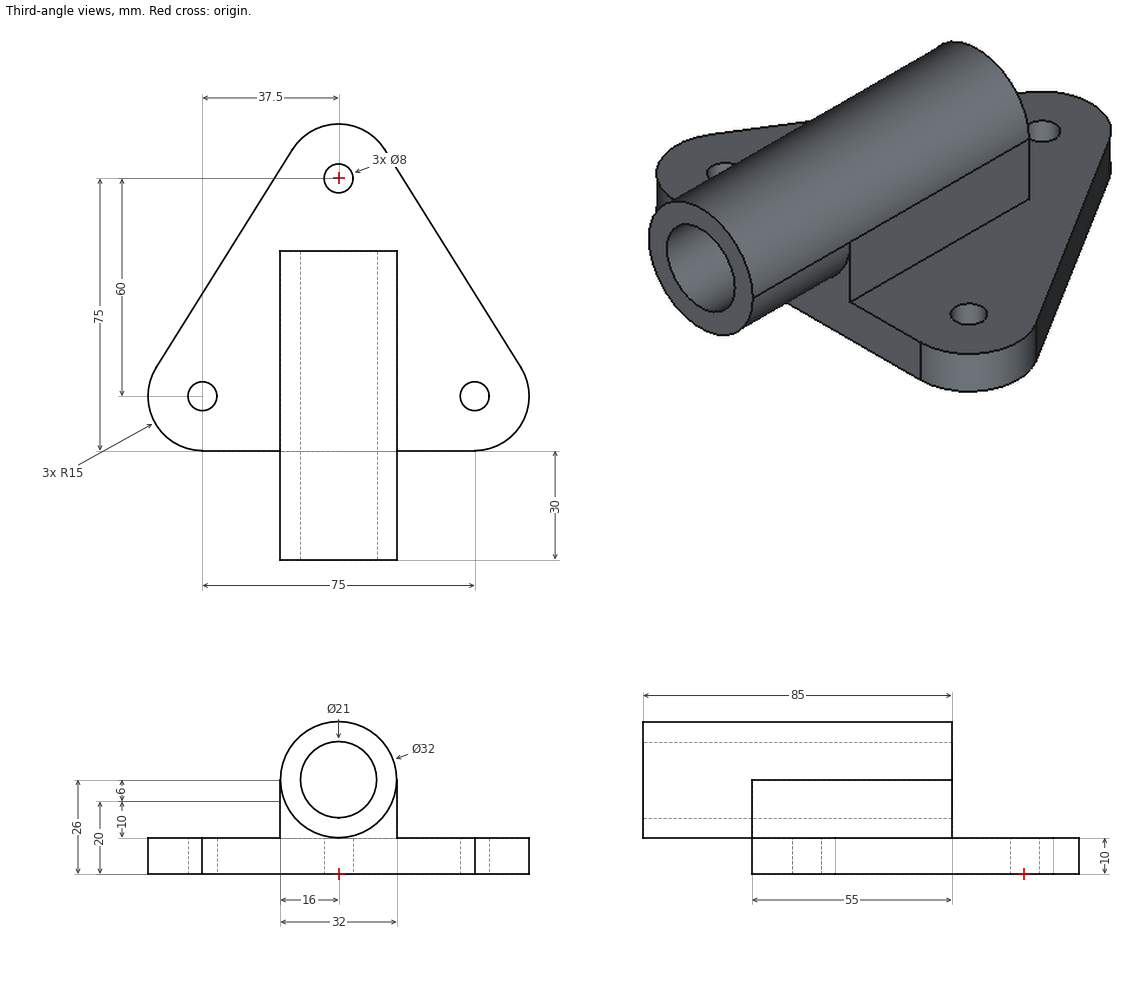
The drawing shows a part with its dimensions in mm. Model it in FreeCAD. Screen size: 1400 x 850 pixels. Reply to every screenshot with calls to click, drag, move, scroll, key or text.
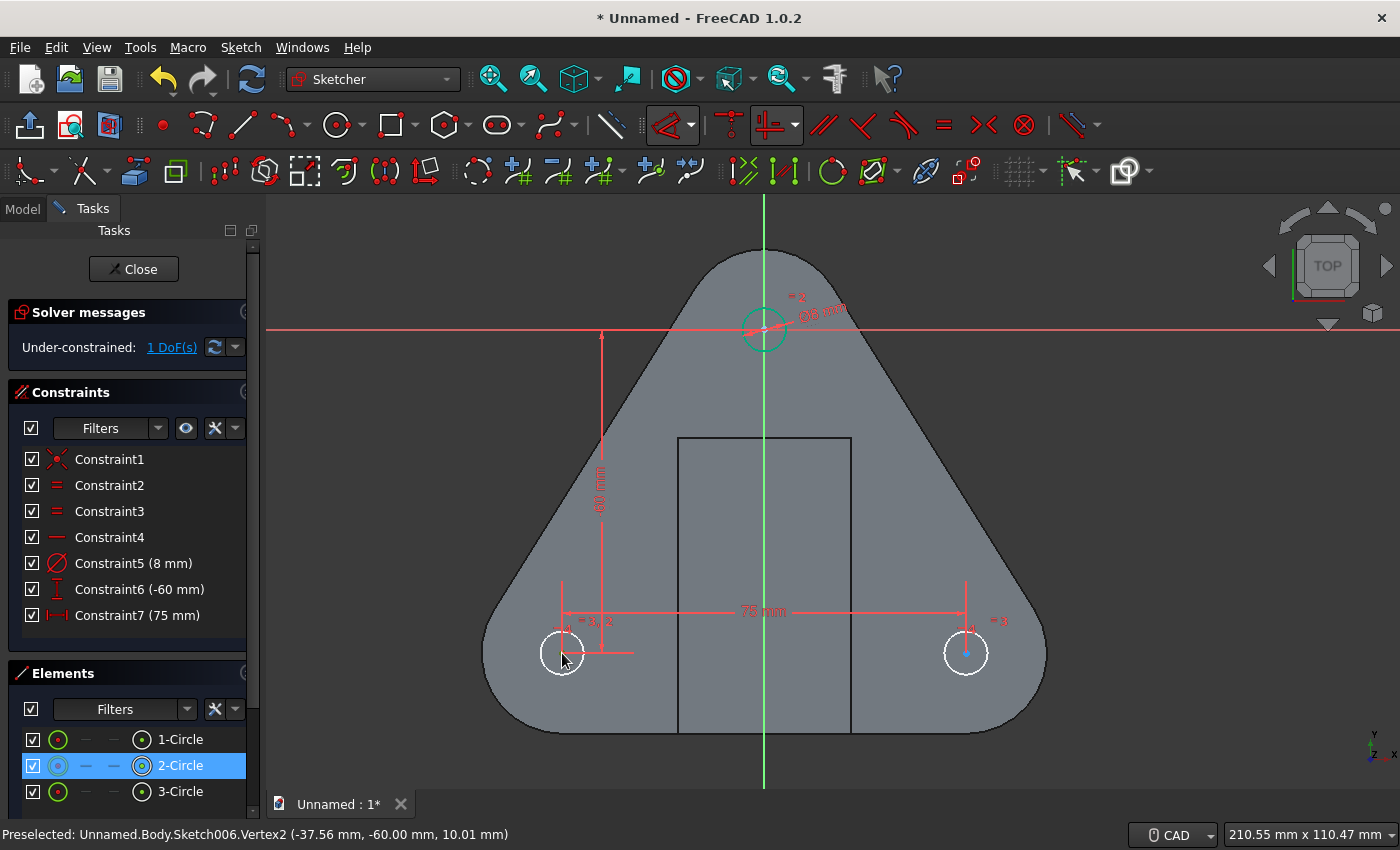
key(l)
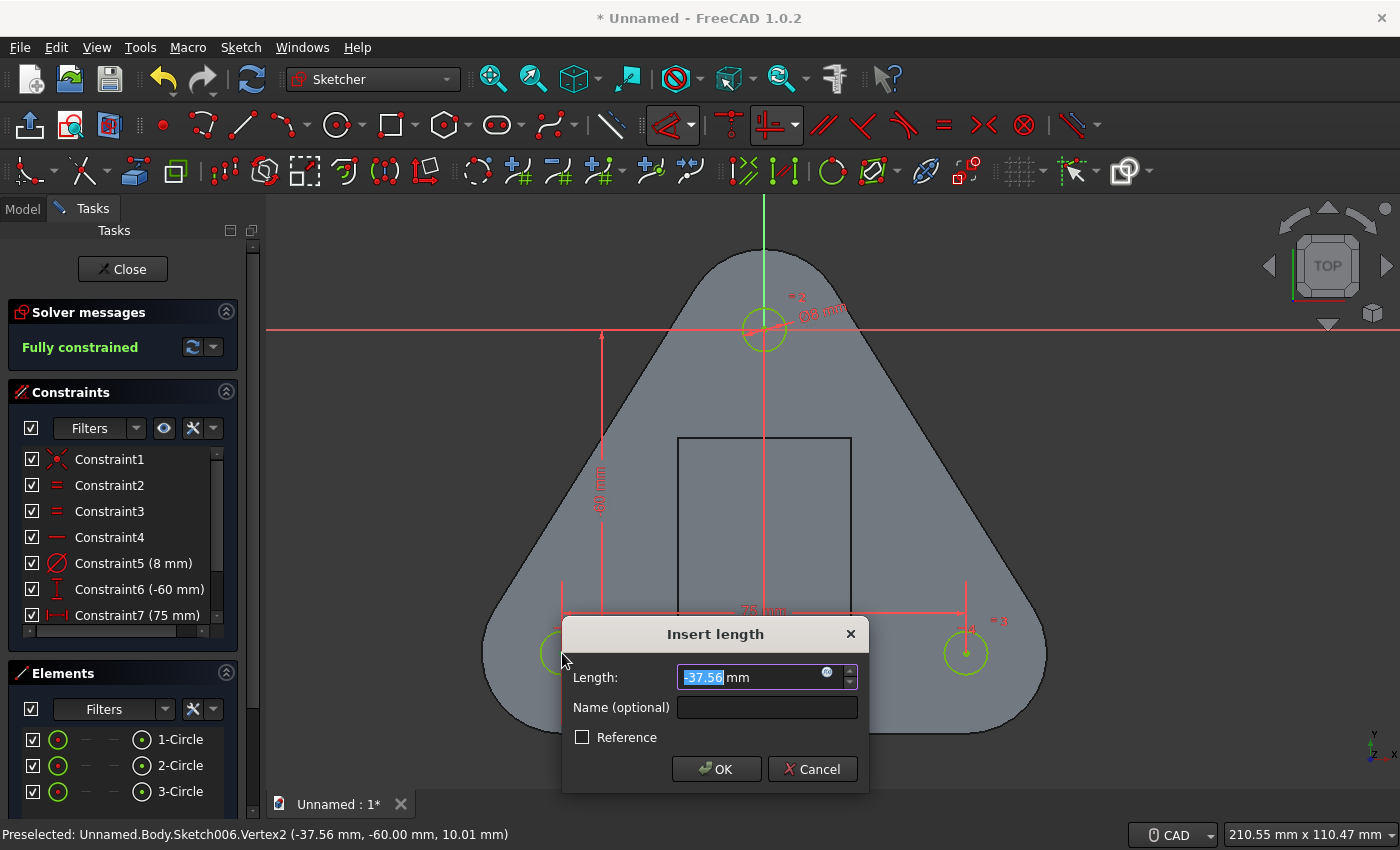
text(-37.5)
key(Return)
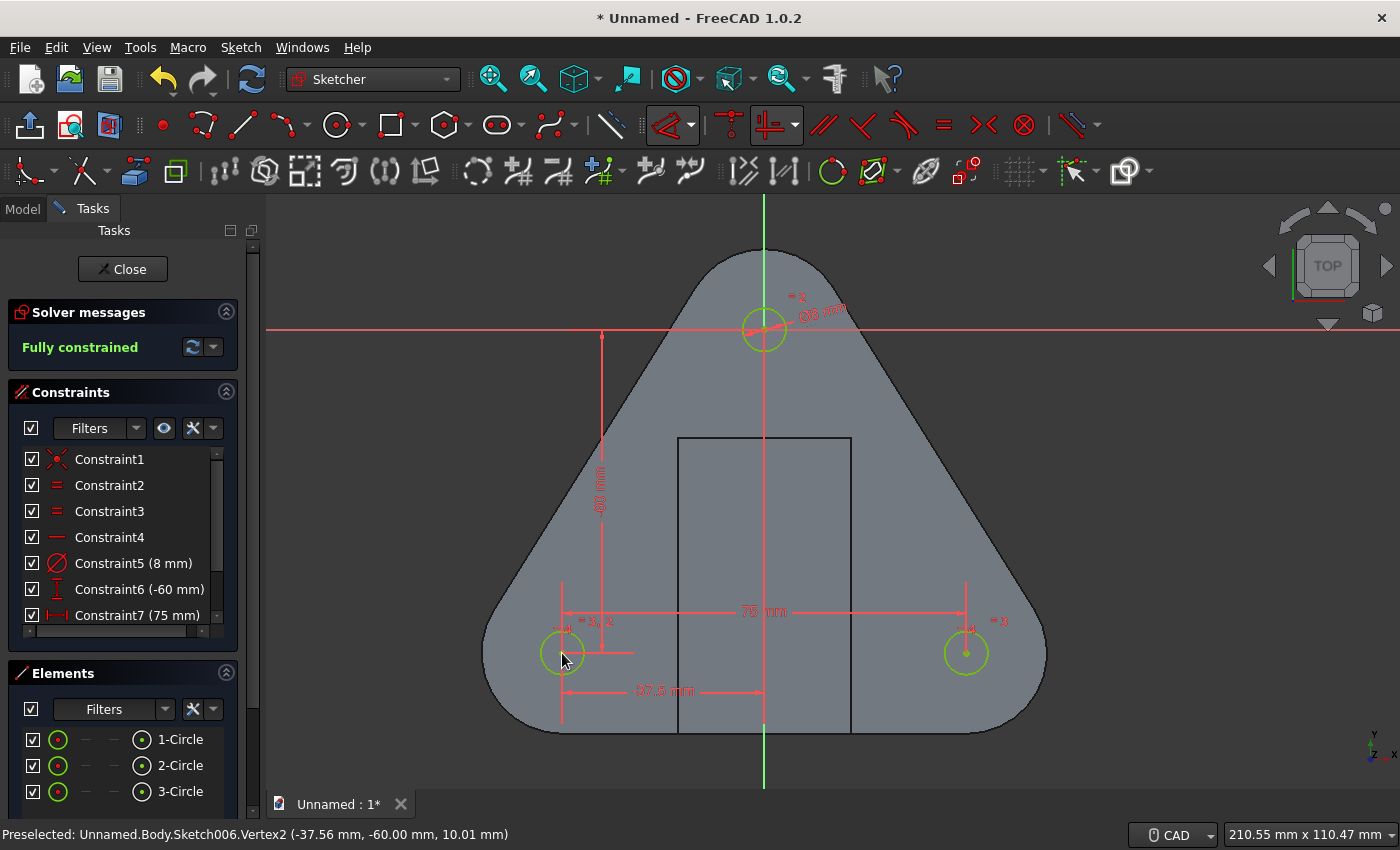
click(123, 269)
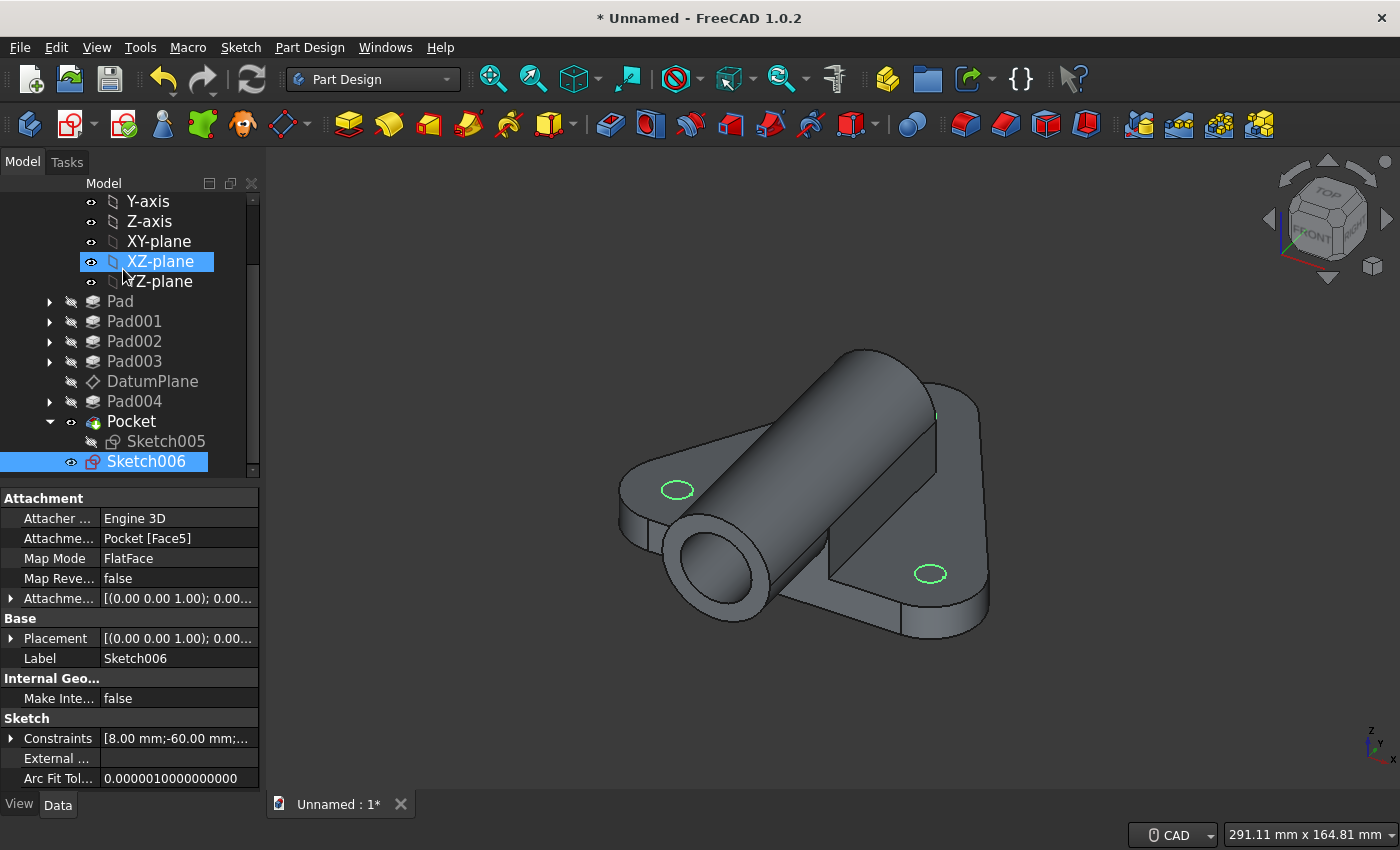
click(612, 124)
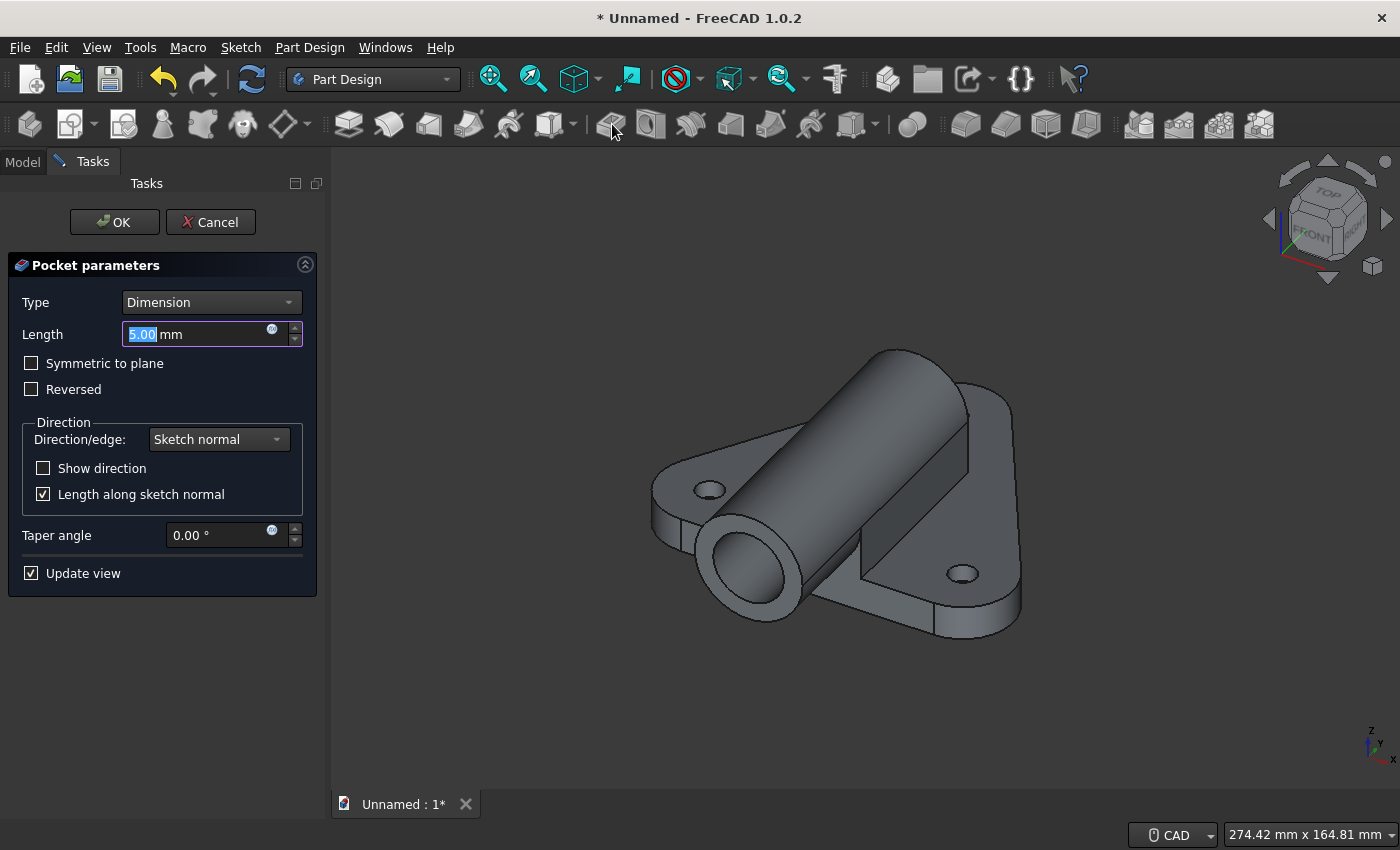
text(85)
key(Tab)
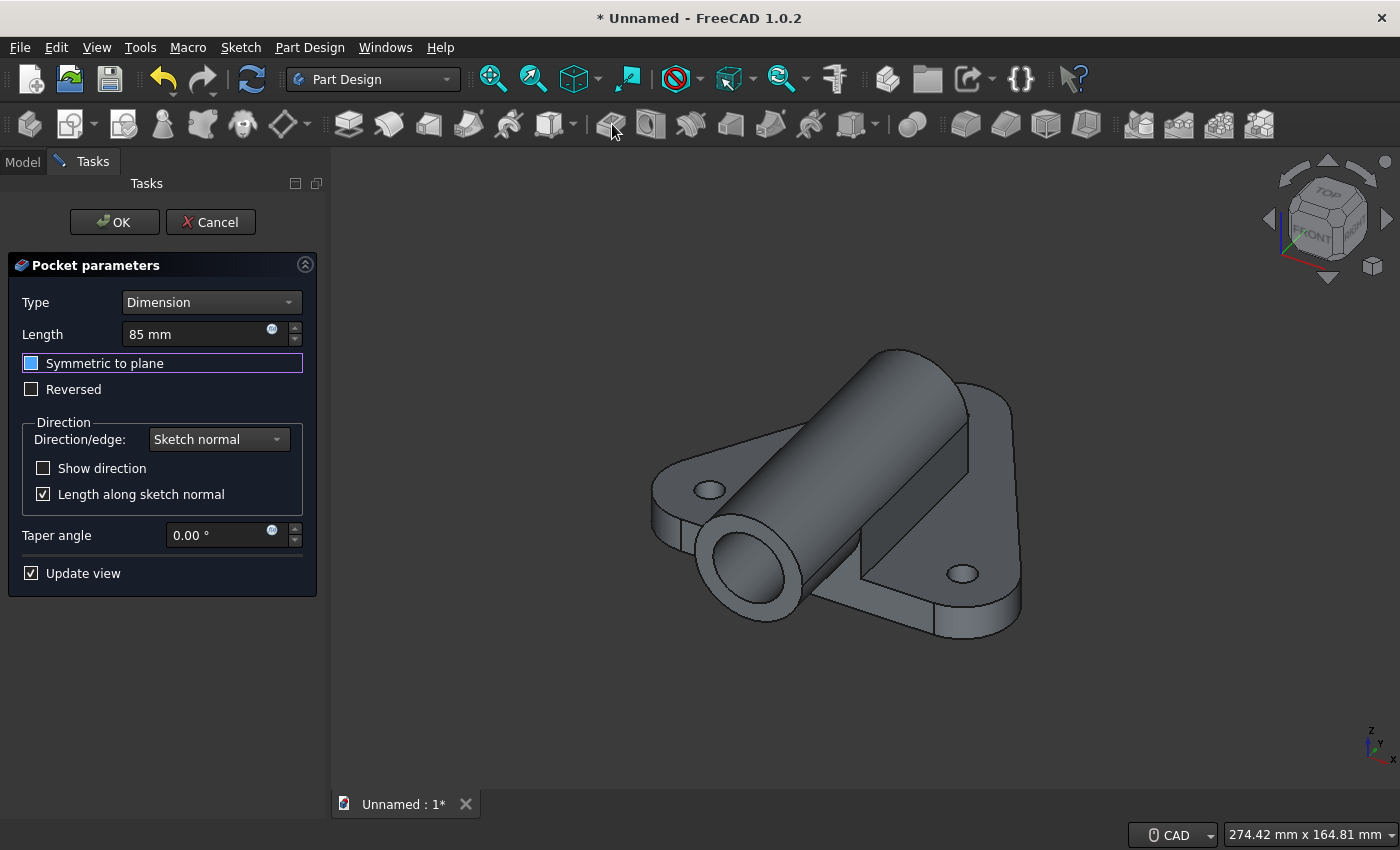
click(115, 222)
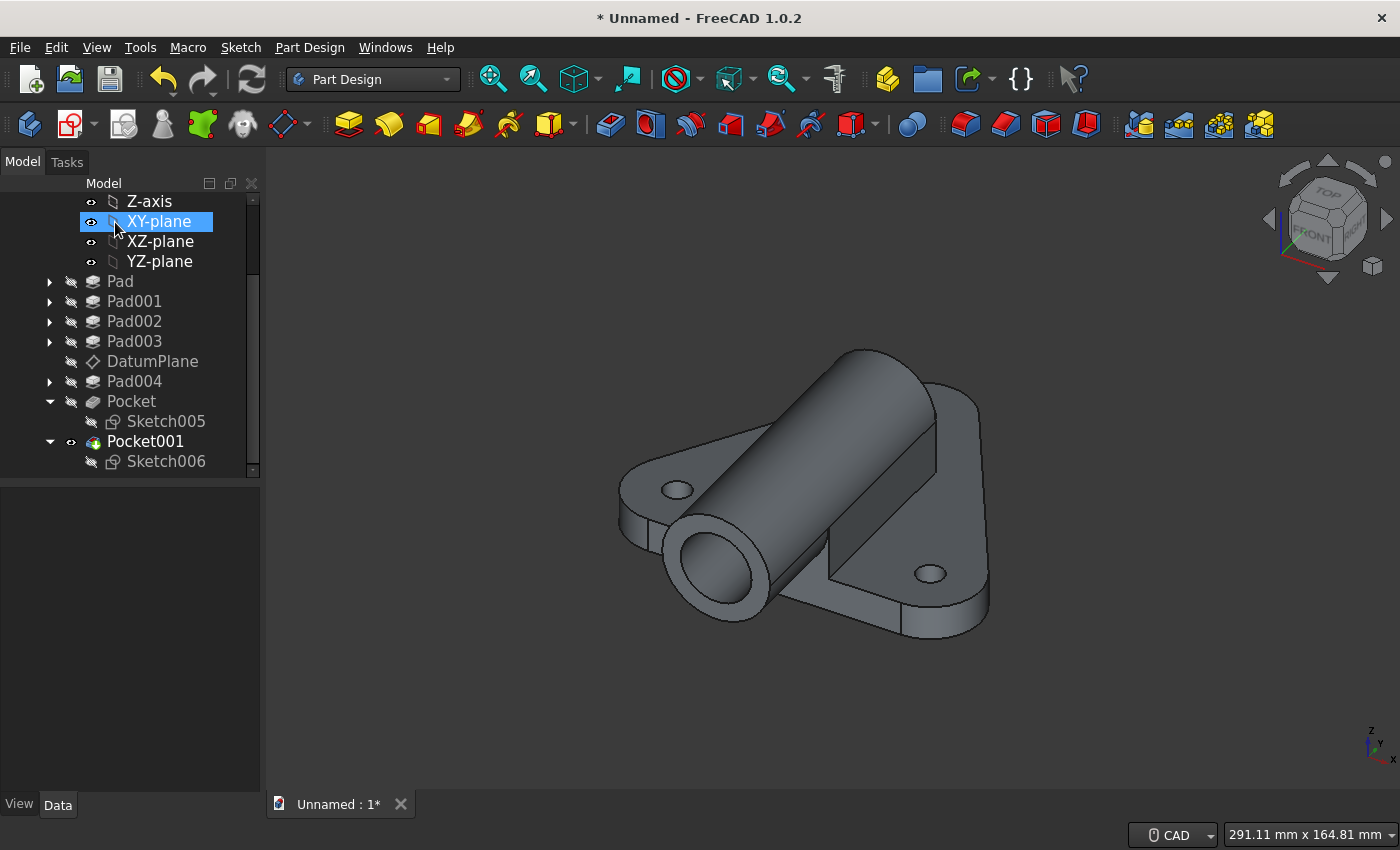
key(0)